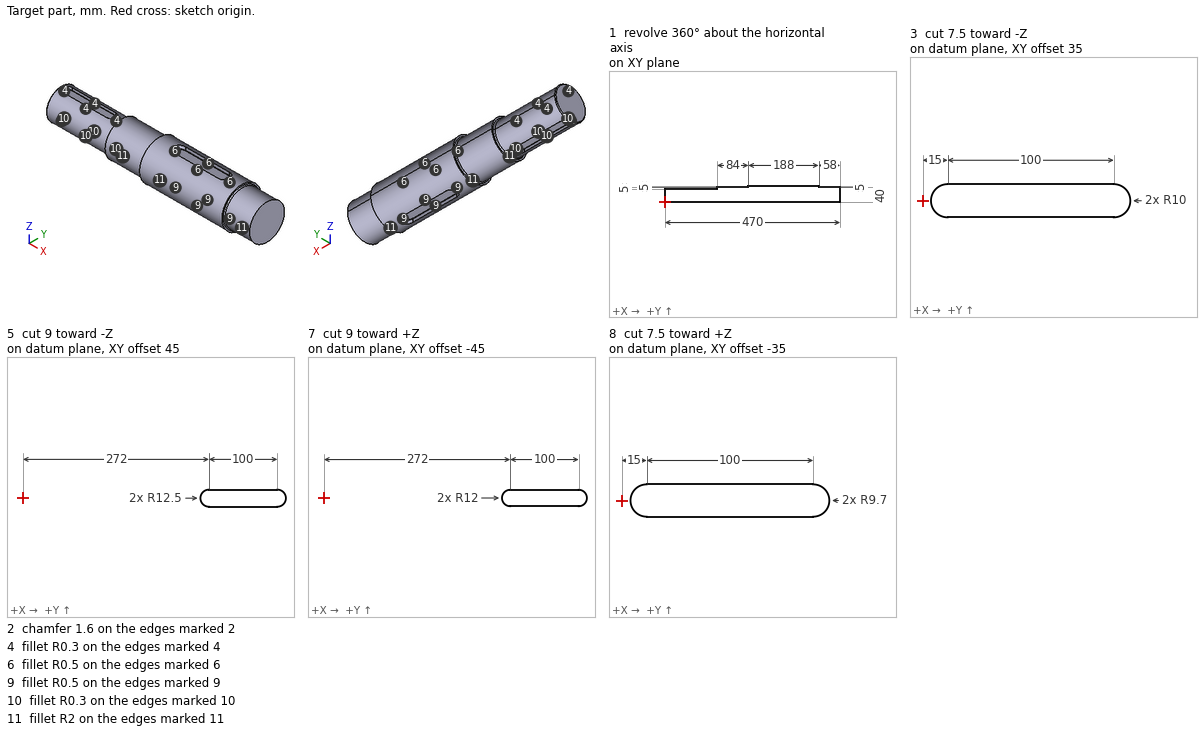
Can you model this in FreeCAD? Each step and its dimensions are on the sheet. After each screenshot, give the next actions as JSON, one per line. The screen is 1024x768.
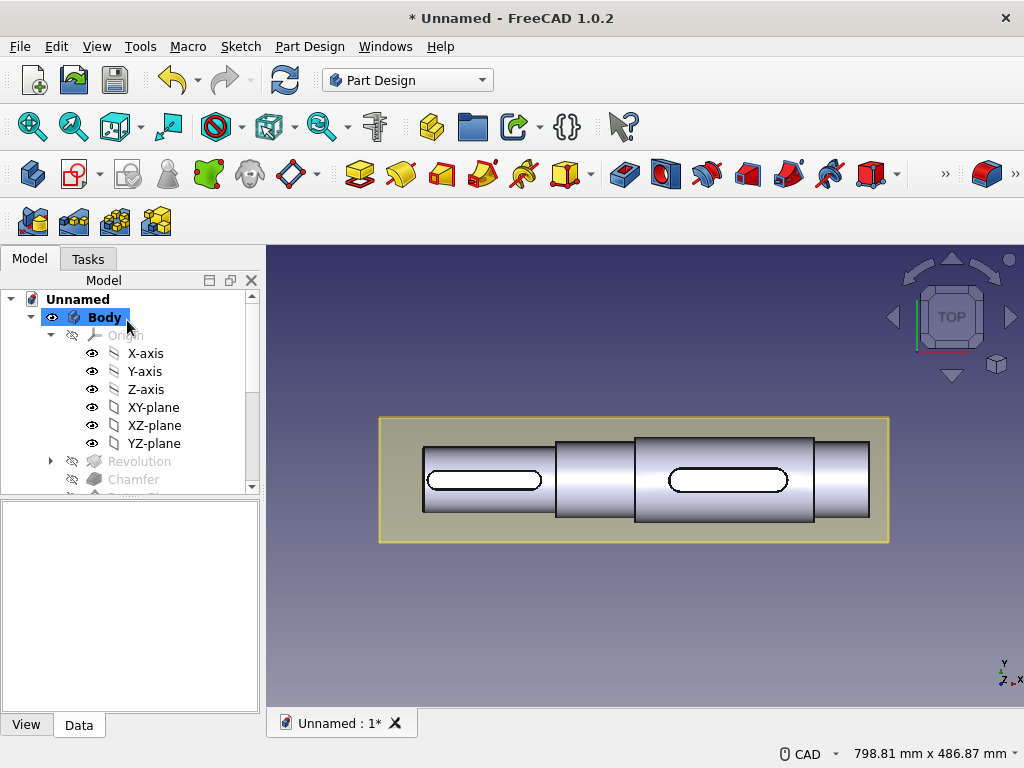
{"action": "scroll", "coordinate": [101, 385], "scroll_direction": "down", "scroll_amount": 3}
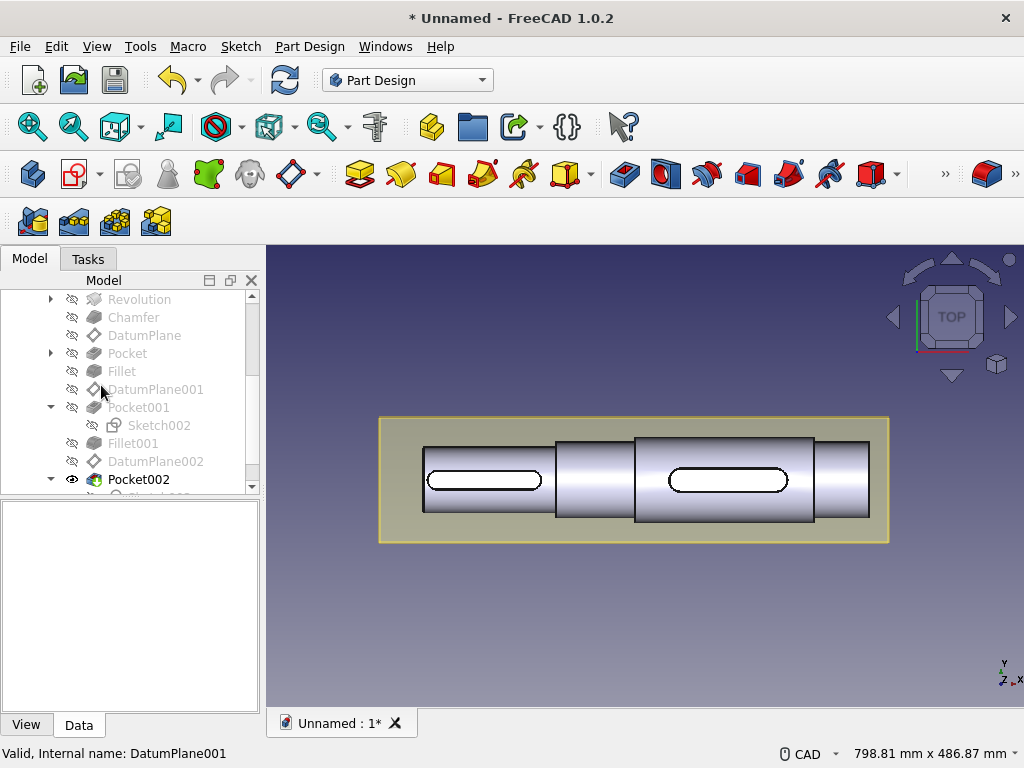
{"action": "scroll", "coordinate": [141, 385], "scroll_direction": "up", "scroll_amount": 15}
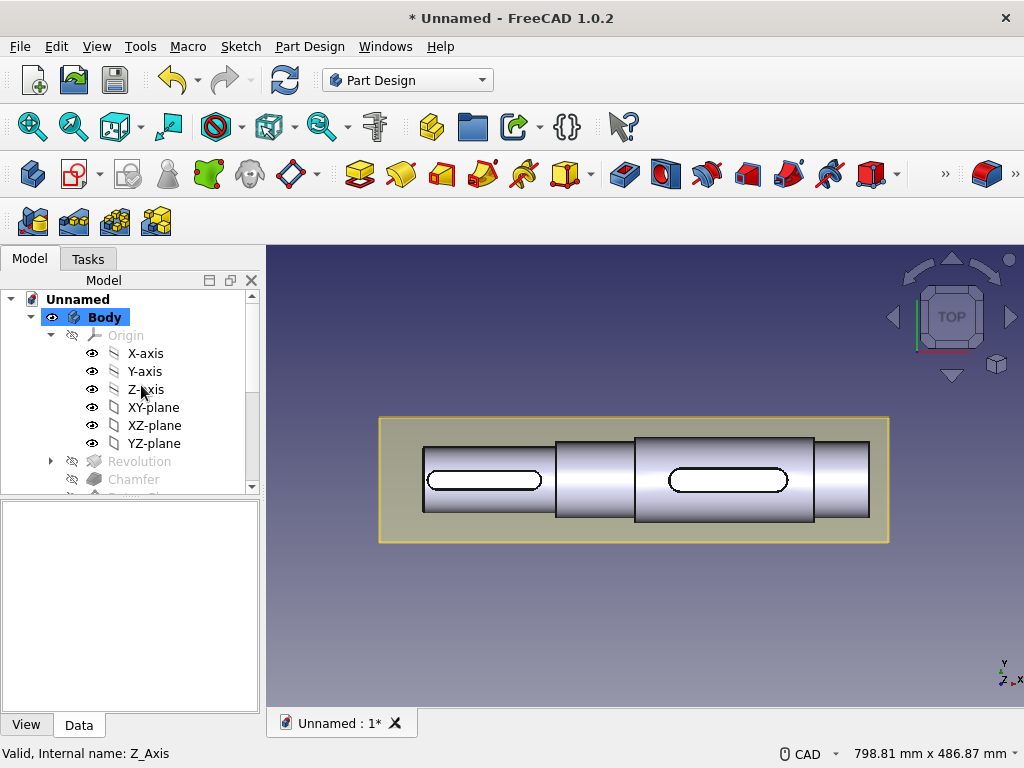
{"action": "scroll", "coordinate": [101, 385], "scroll_direction": "down", "scroll_amount": 6}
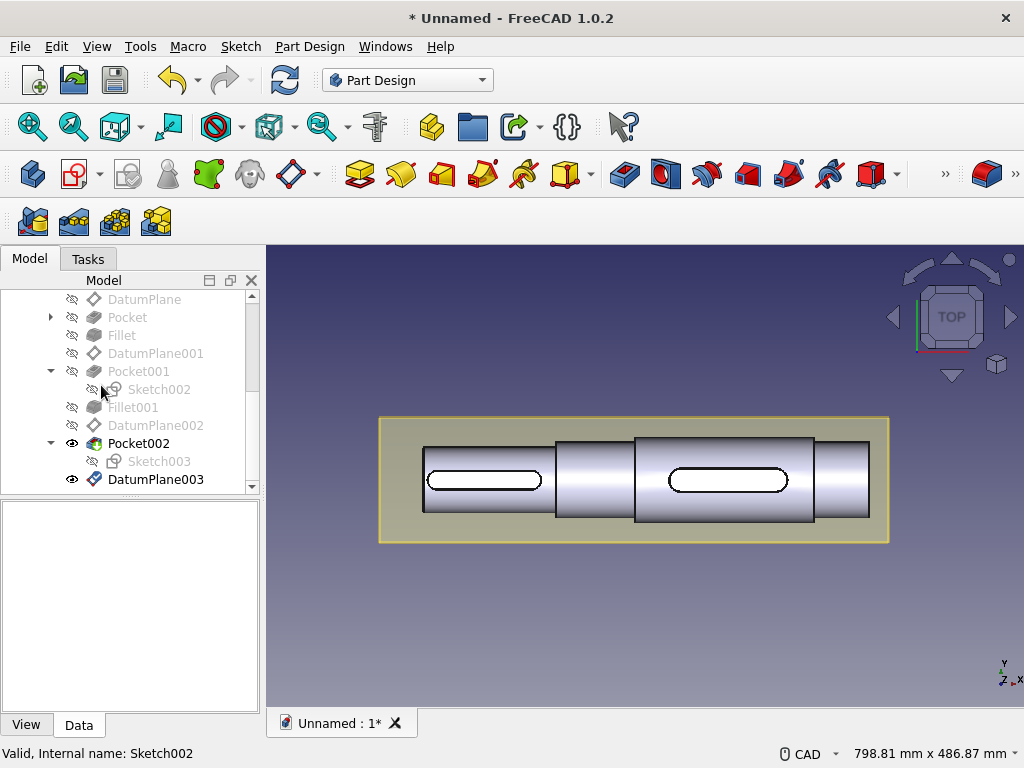
{"action": "left_click", "coordinate": [117, 479]}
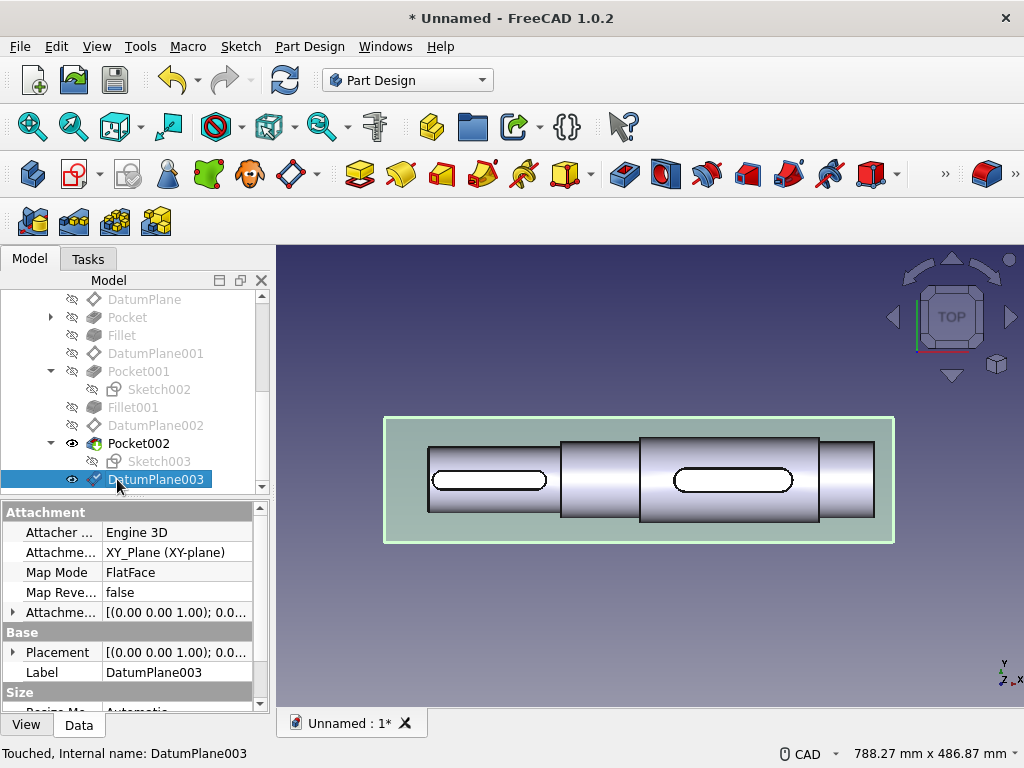
{"action": "left_click", "coordinate": [74, 174]}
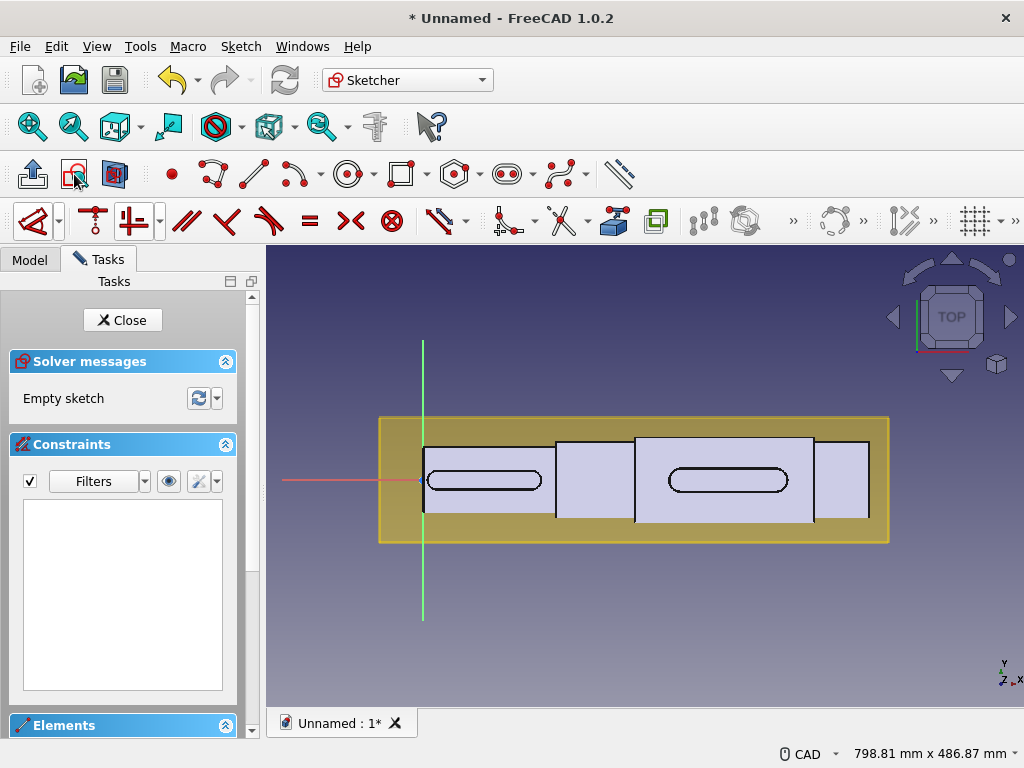
{"action": "left_click", "coordinate": [115, 174]}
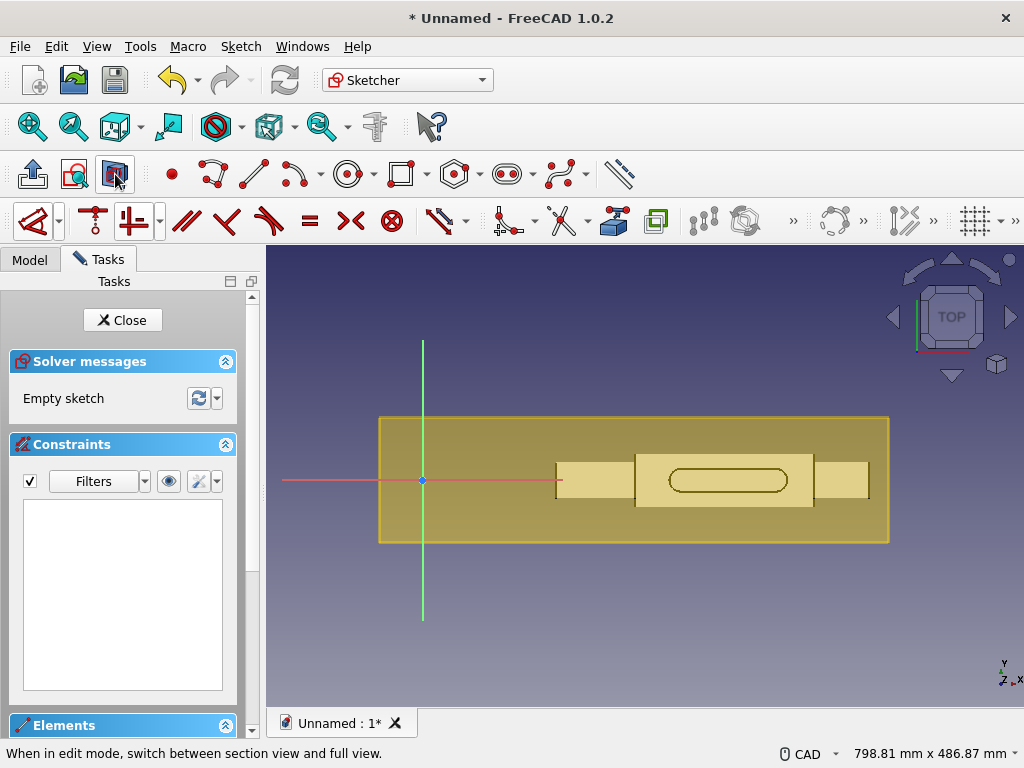
{"action": "scroll", "coordinate": [441, 482], "scroll_direction": "up", "scroll_amount": 6}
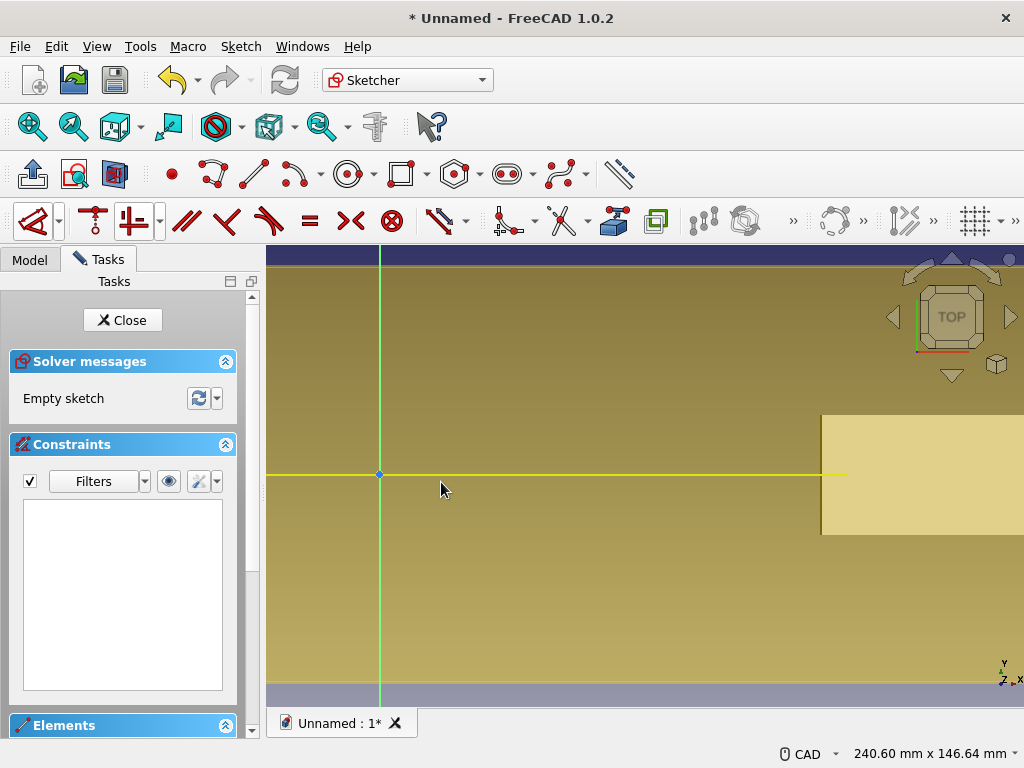
{"action": "left_click", "coordinate": [506, 174]}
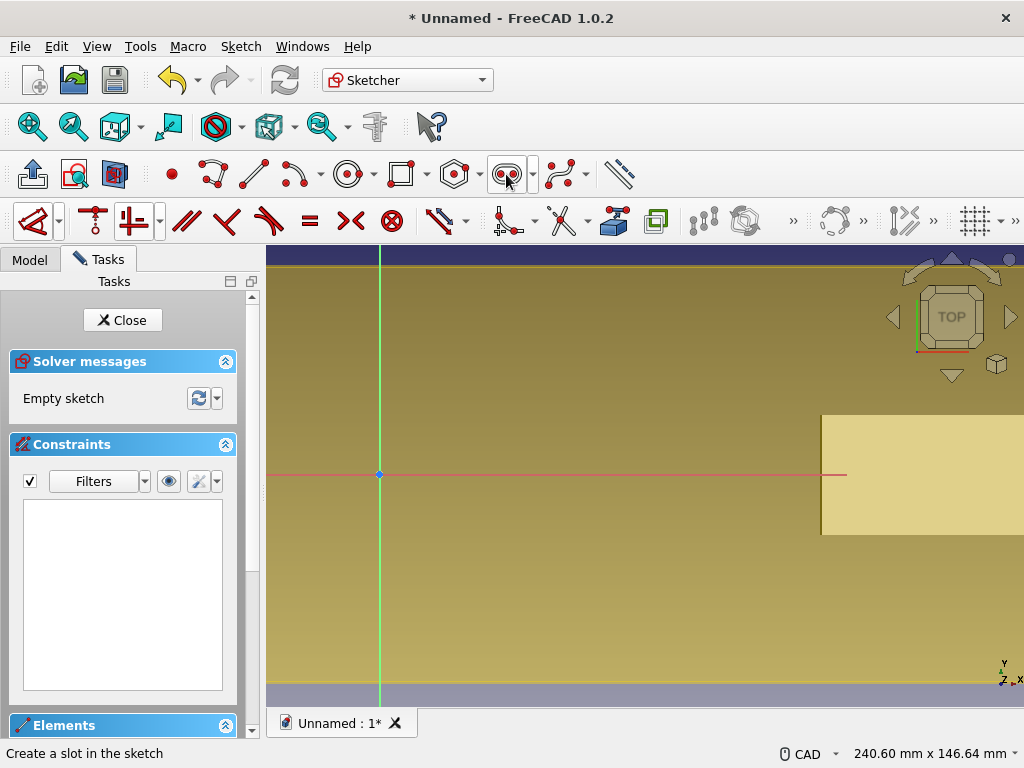
{"action": "left_click", "coordinate": [427, 475]}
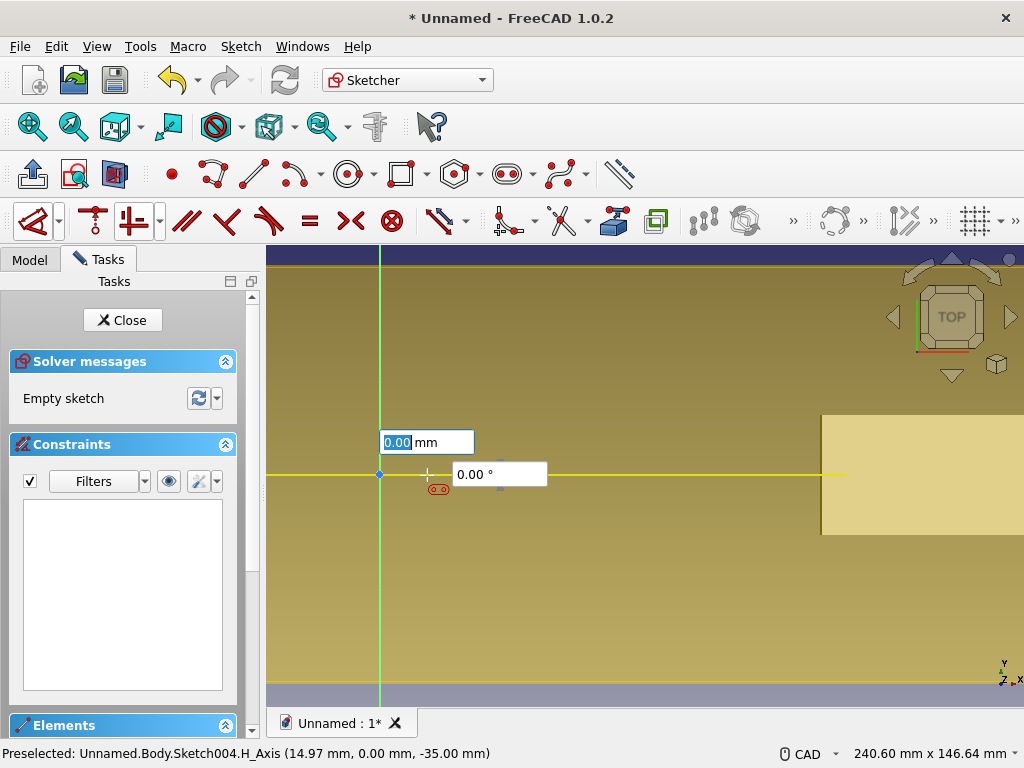
{"action": "left_click", "coordinate": [742, 466]}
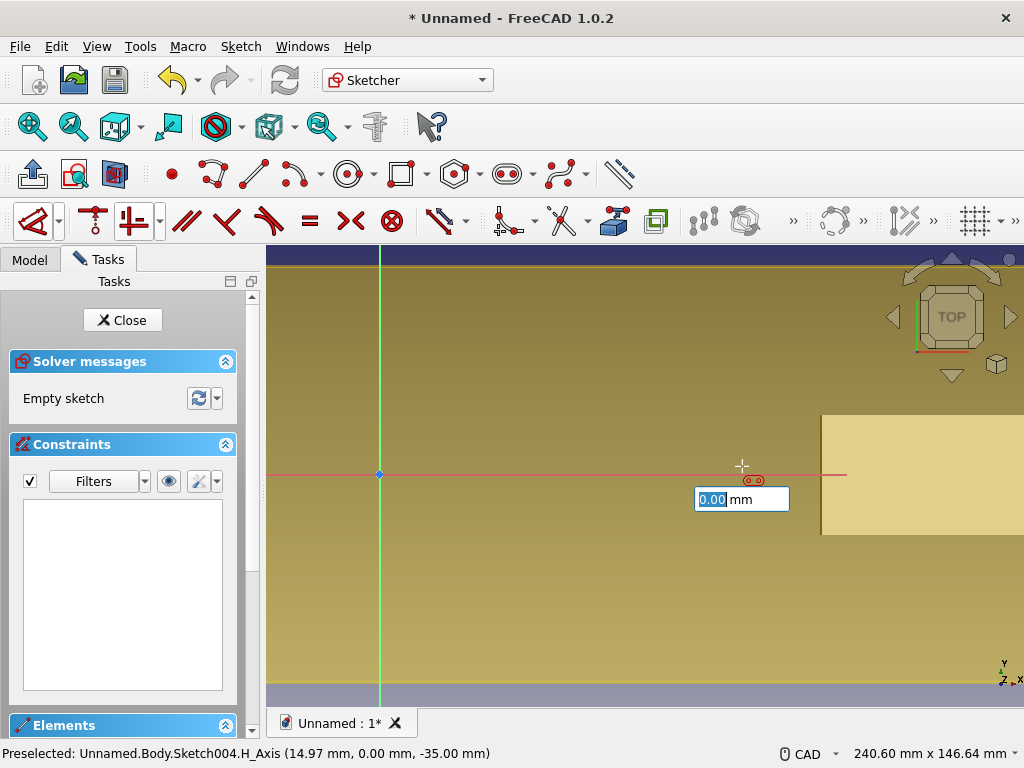
{"action": "left_click", "coordinate": [585, 444]}
{"action": "key", "text": "Escape"}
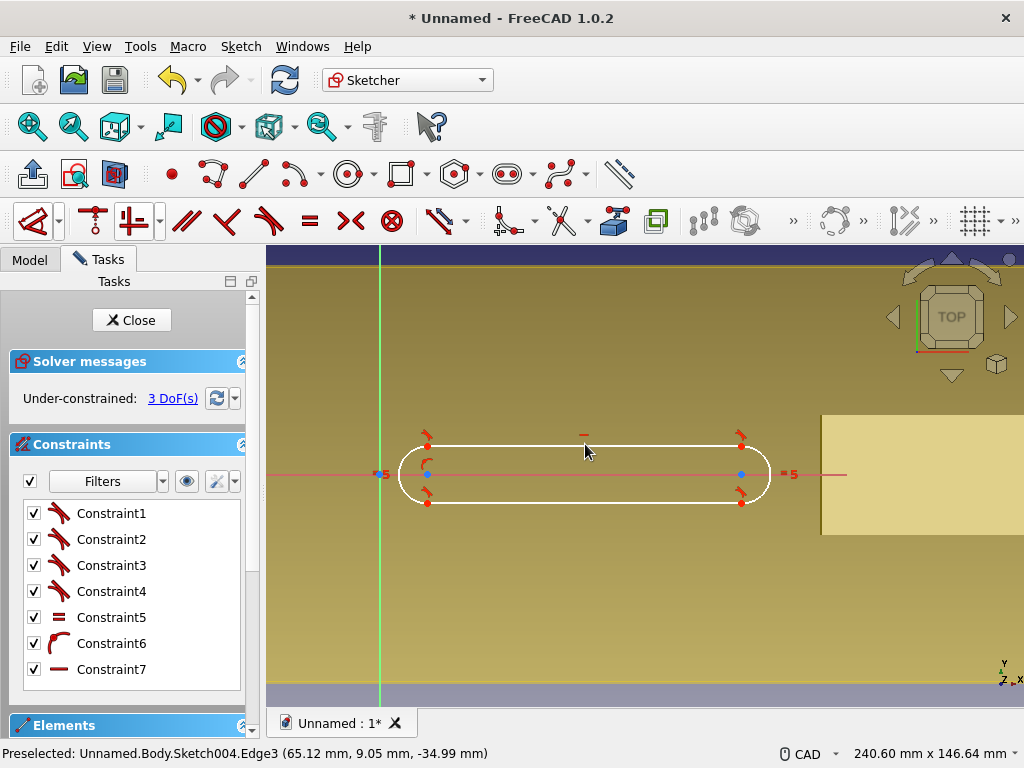
{"action": "scroll", "coordinate": [404, 458], "scroll_direction": "up", "scroll_amount": 2}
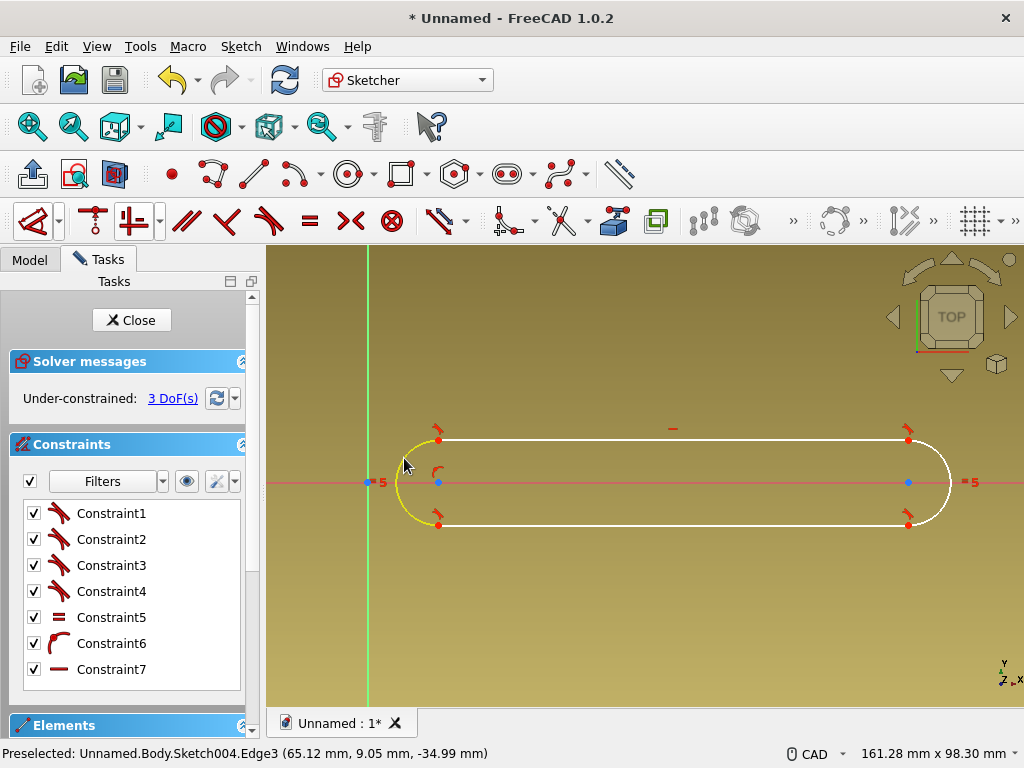
{"action": "left_click", "coordinate": [404, 458]}